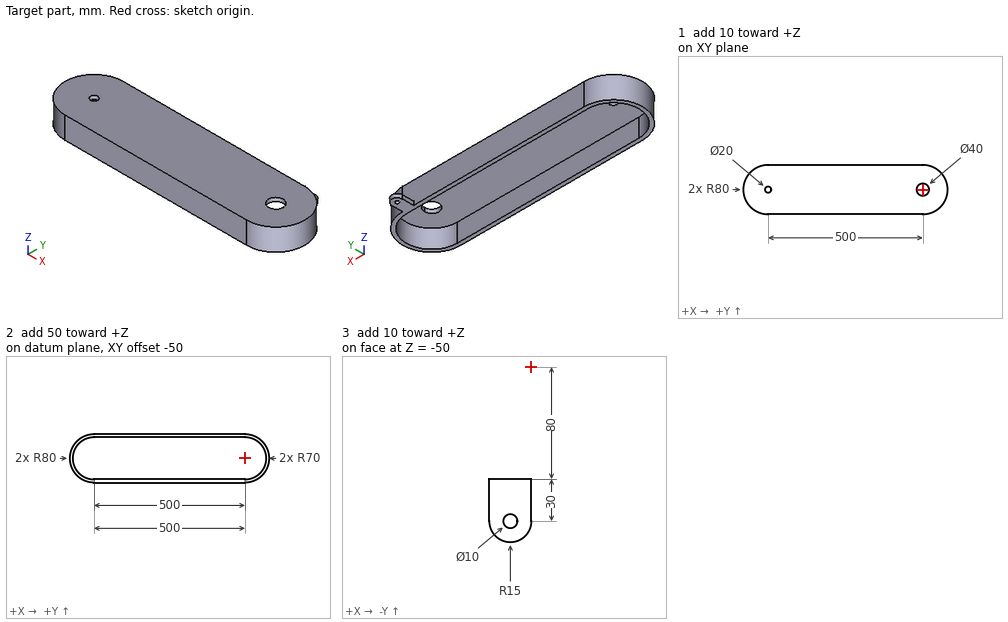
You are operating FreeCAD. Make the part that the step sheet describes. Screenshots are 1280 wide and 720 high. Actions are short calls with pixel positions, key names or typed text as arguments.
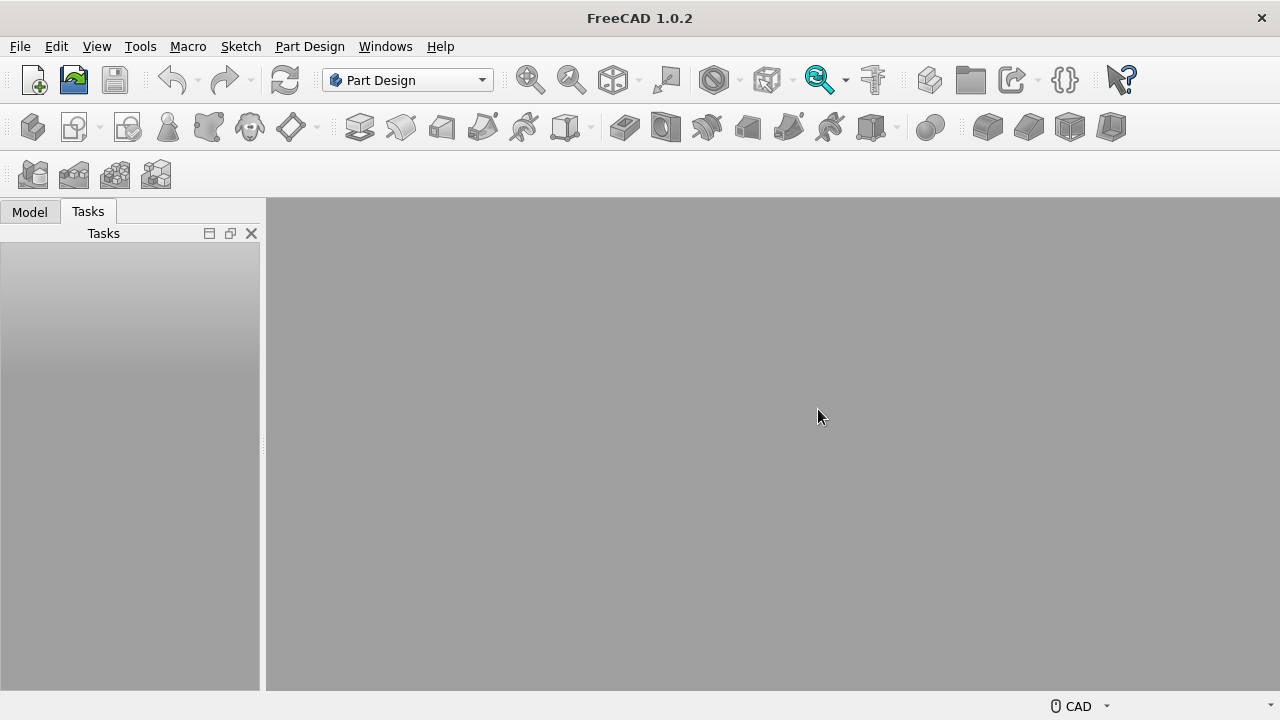
key(ctrl+n)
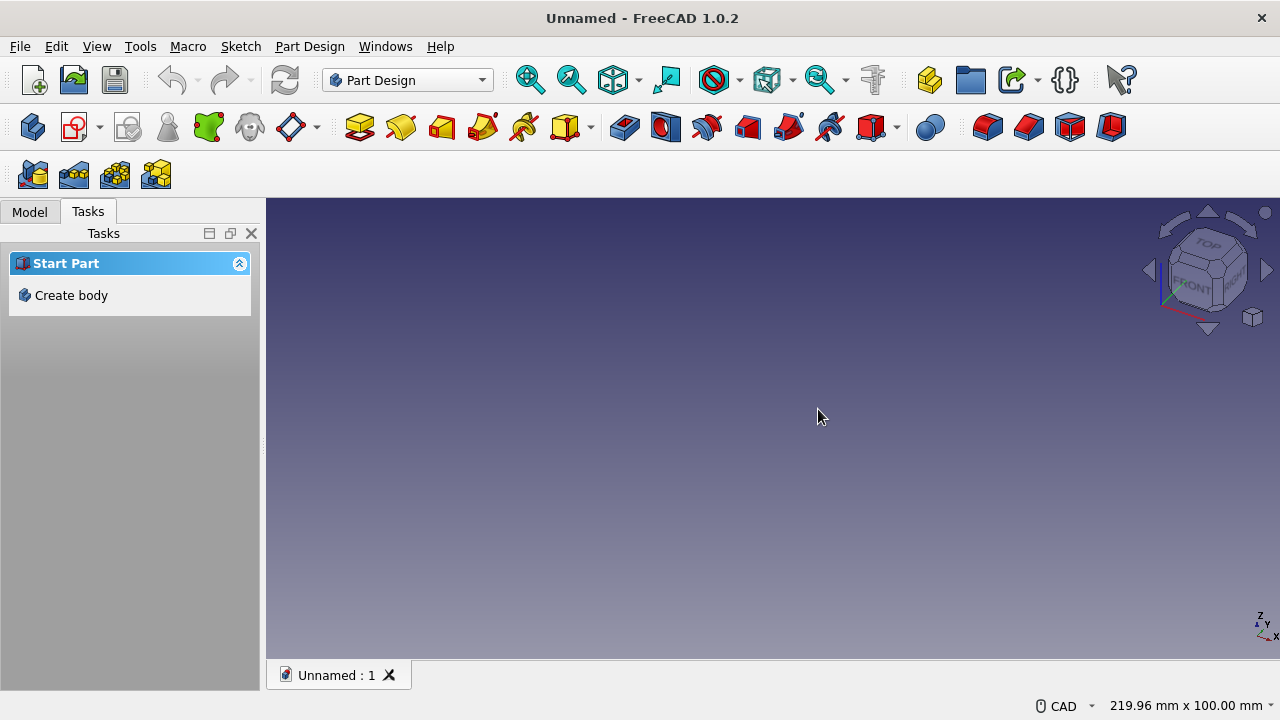
click(74, 128)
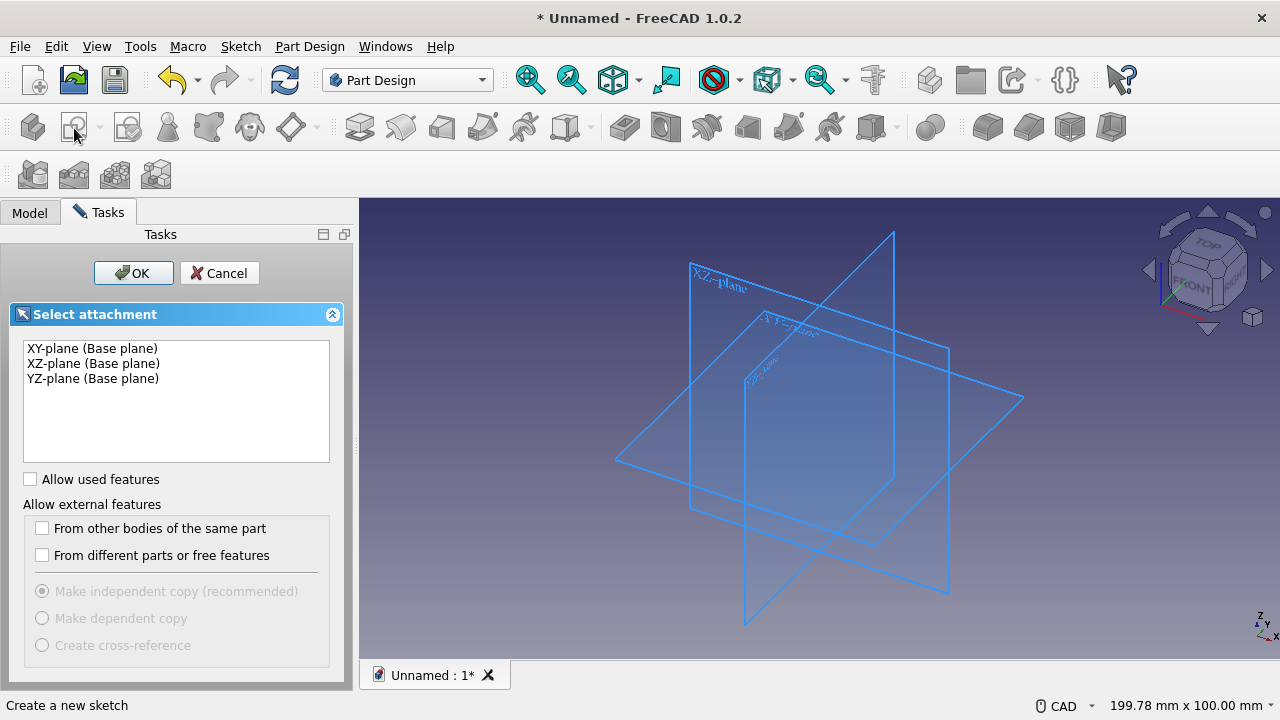
click(84, 348)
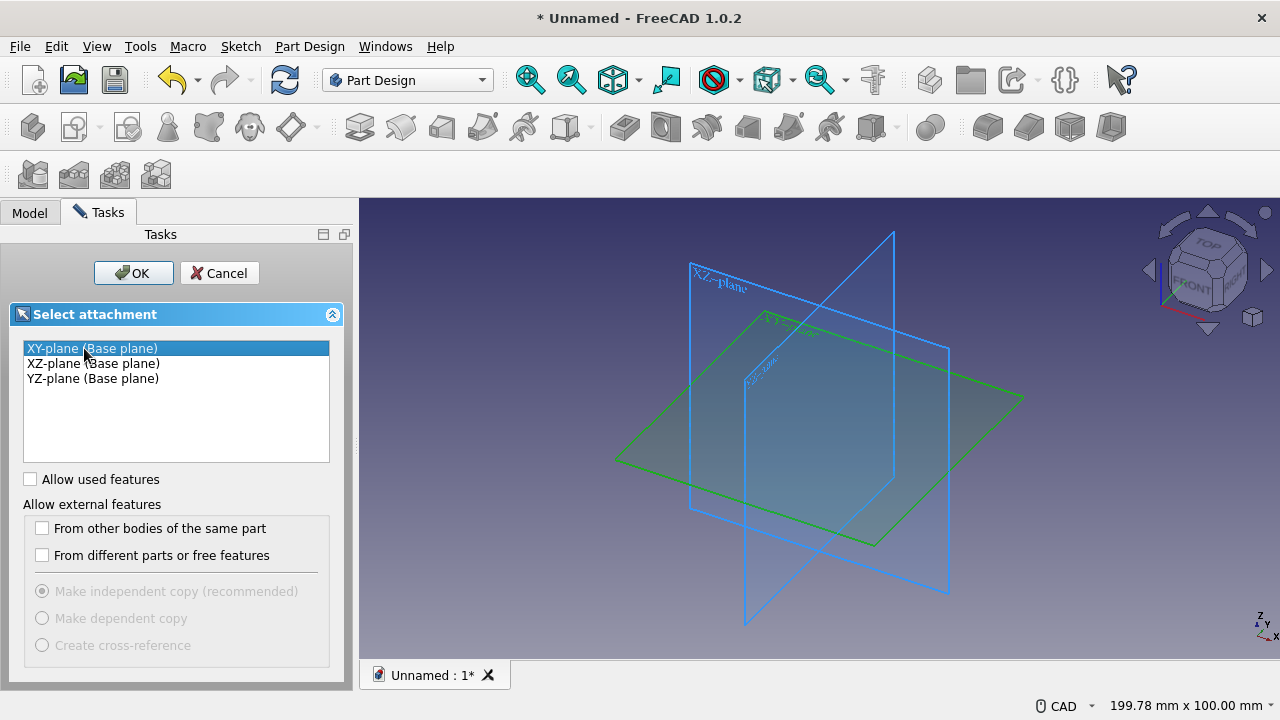
click(134, 273)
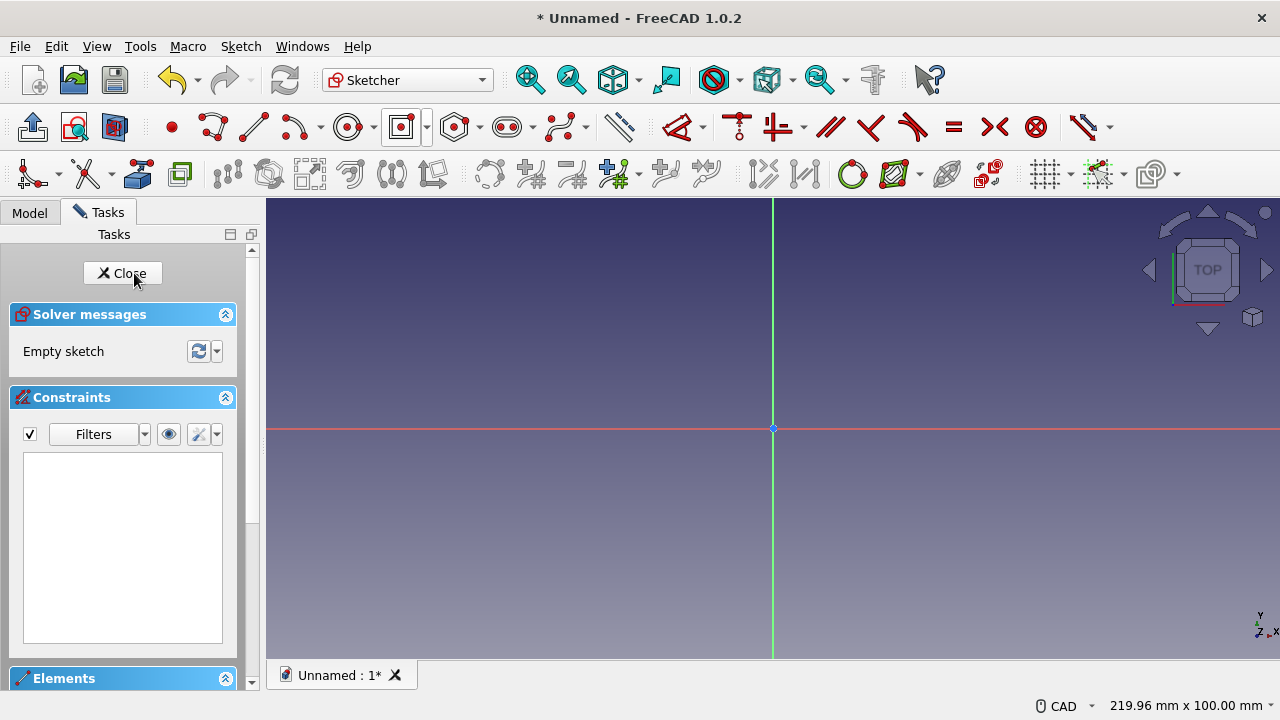
scroll(979, 428, down, 8)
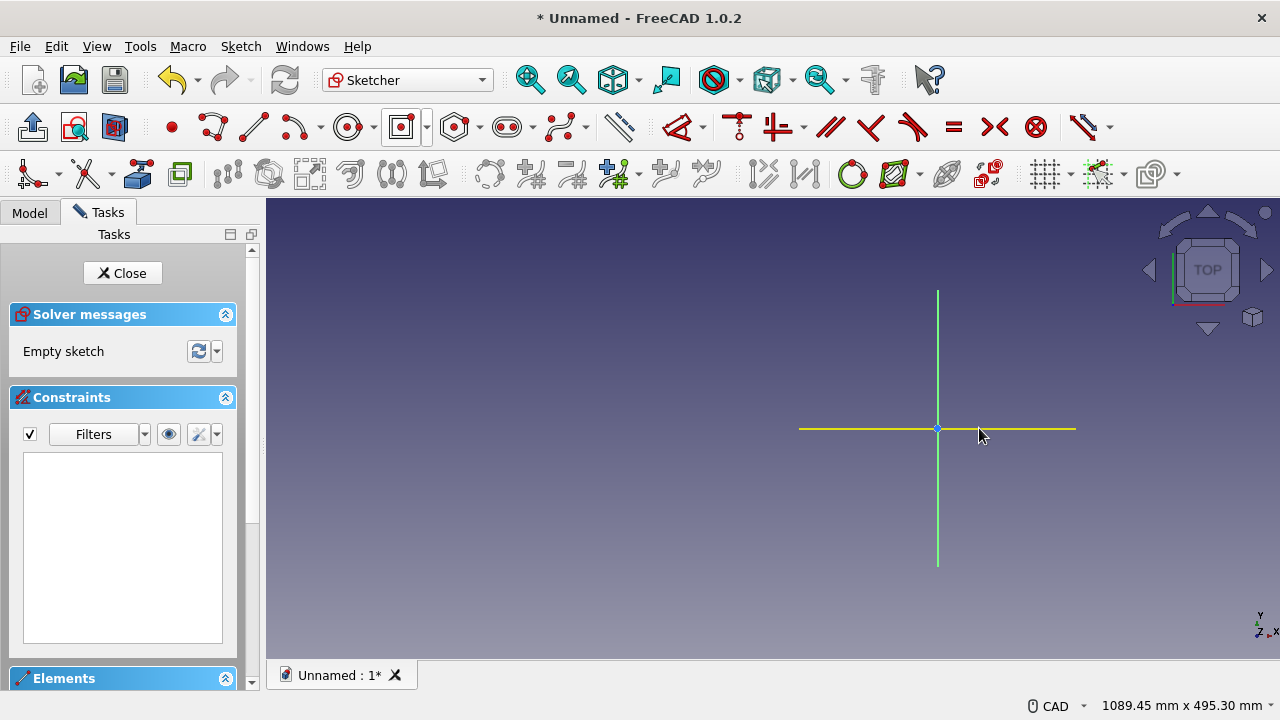
key(g)
key(s)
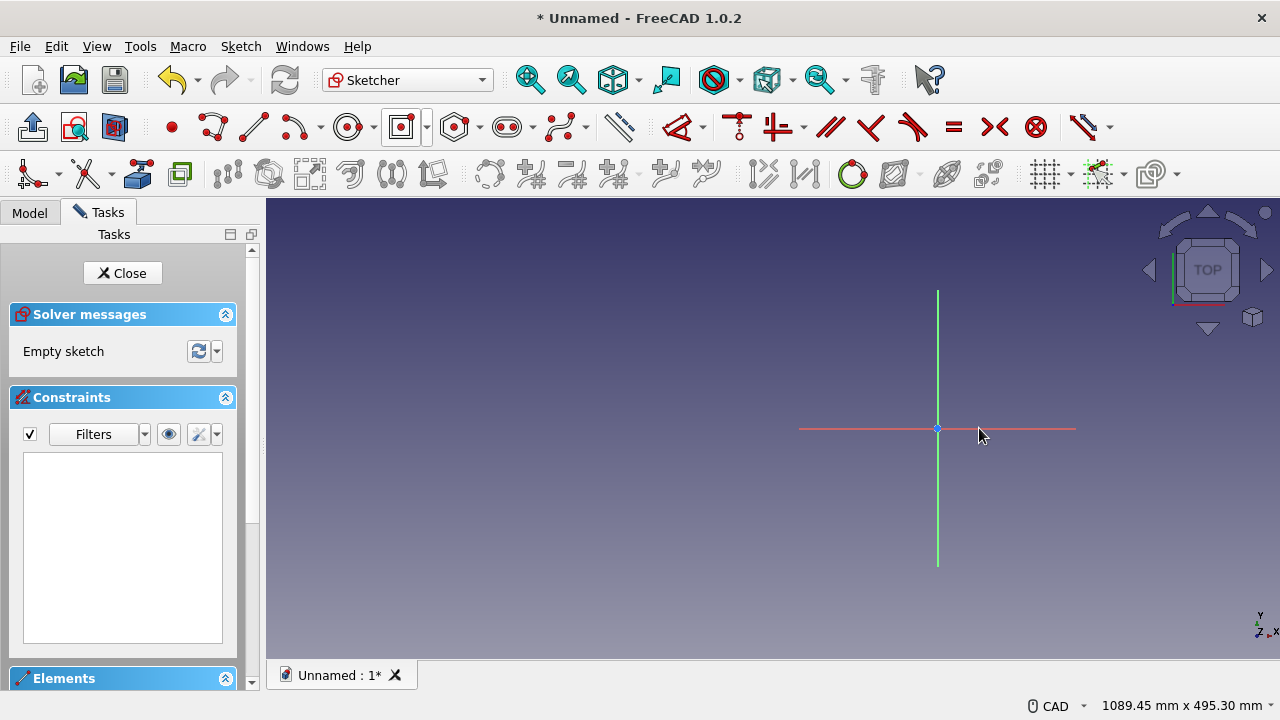
click(938, 428)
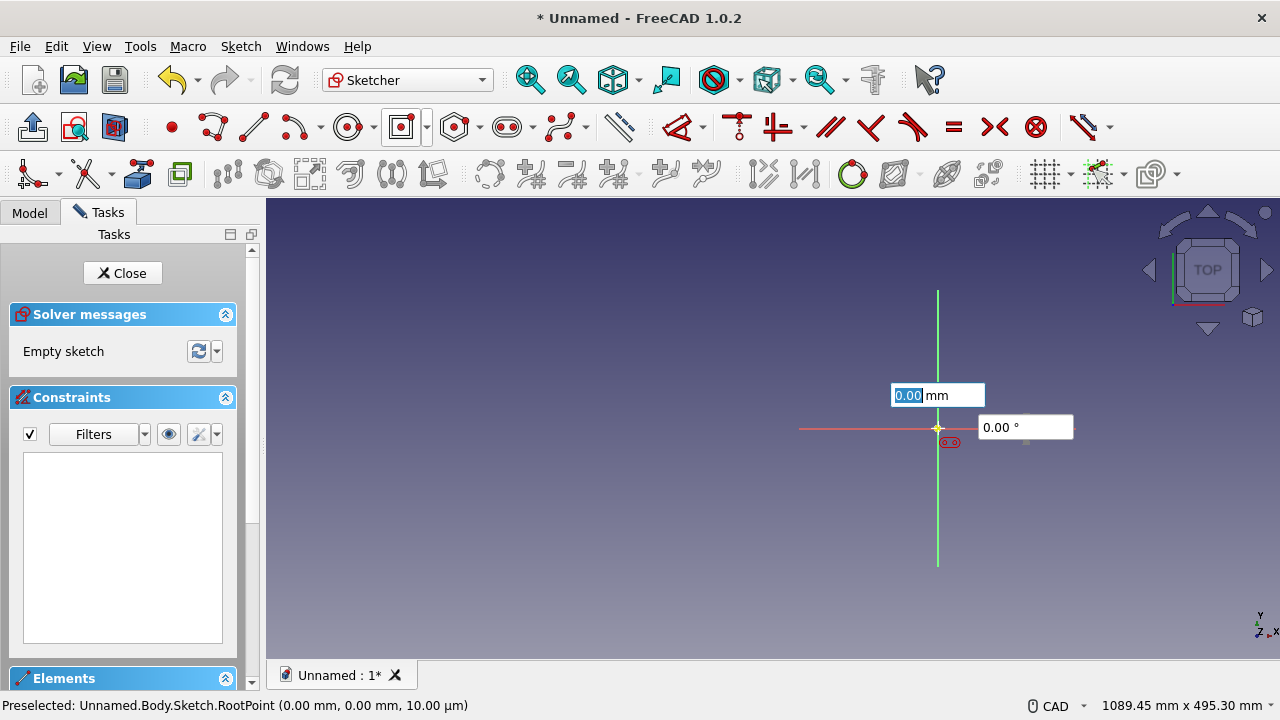
click(473, 420)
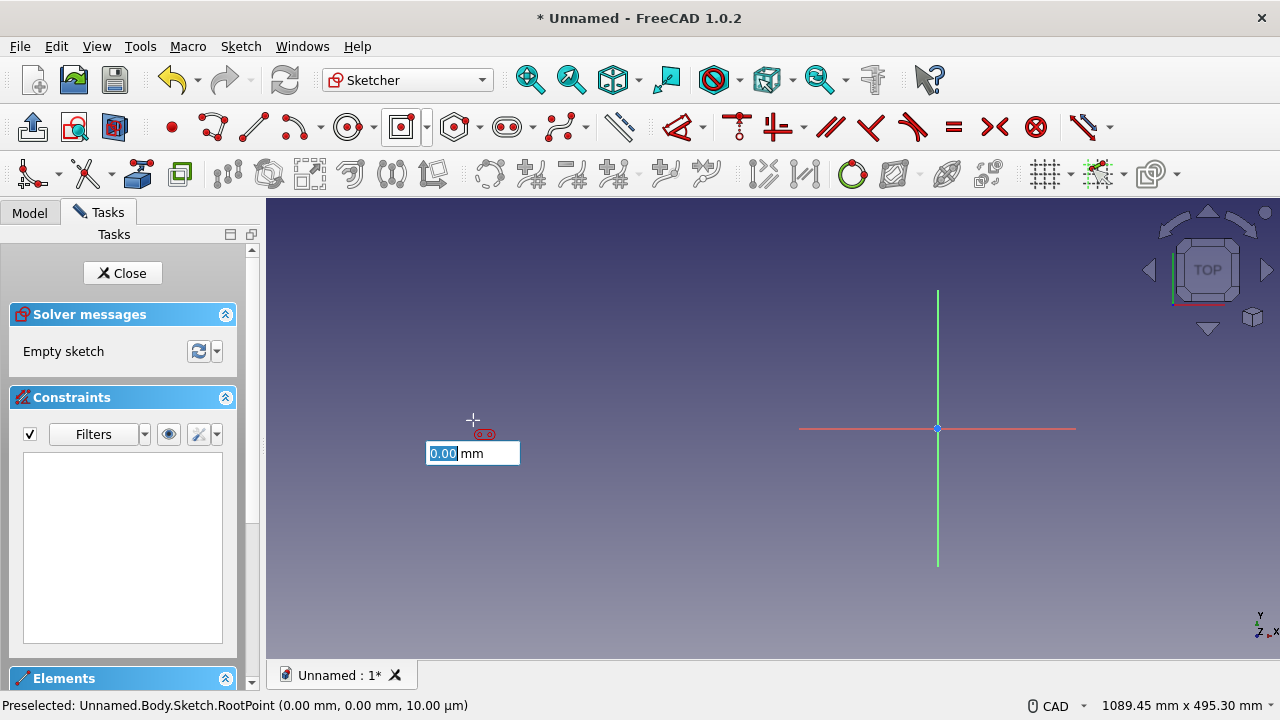
click(705, 354)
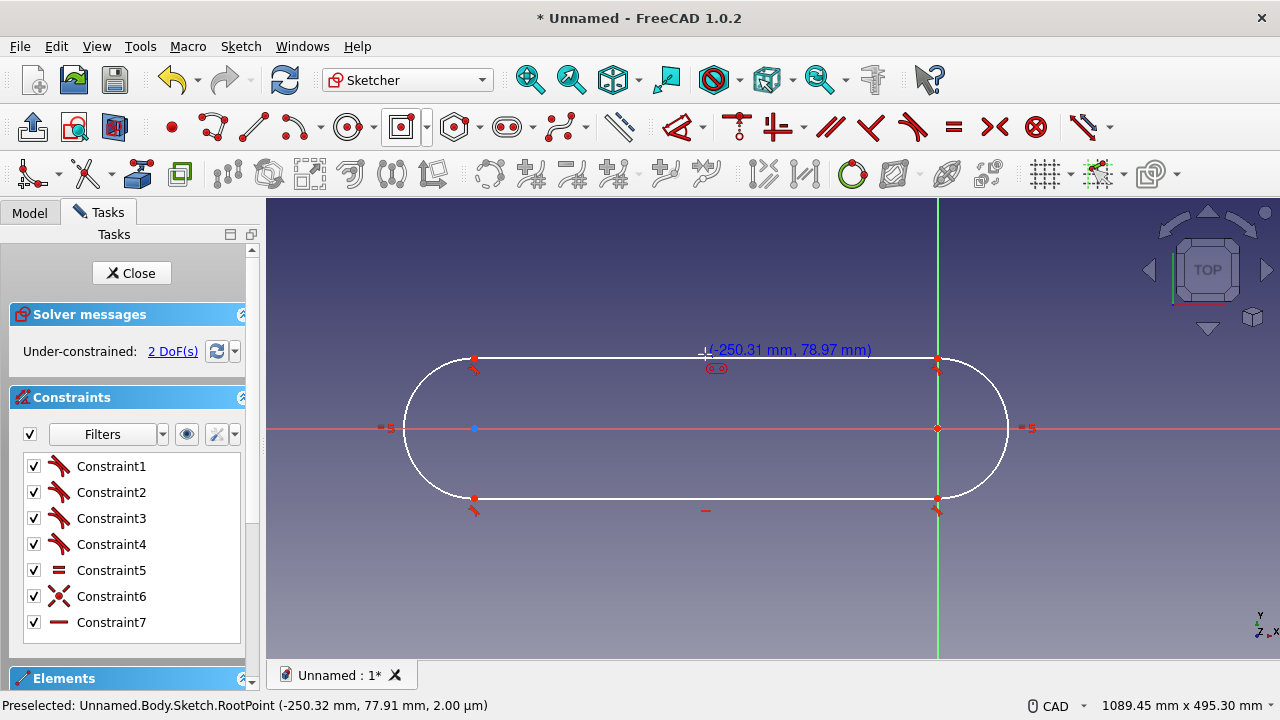
click(348, 128)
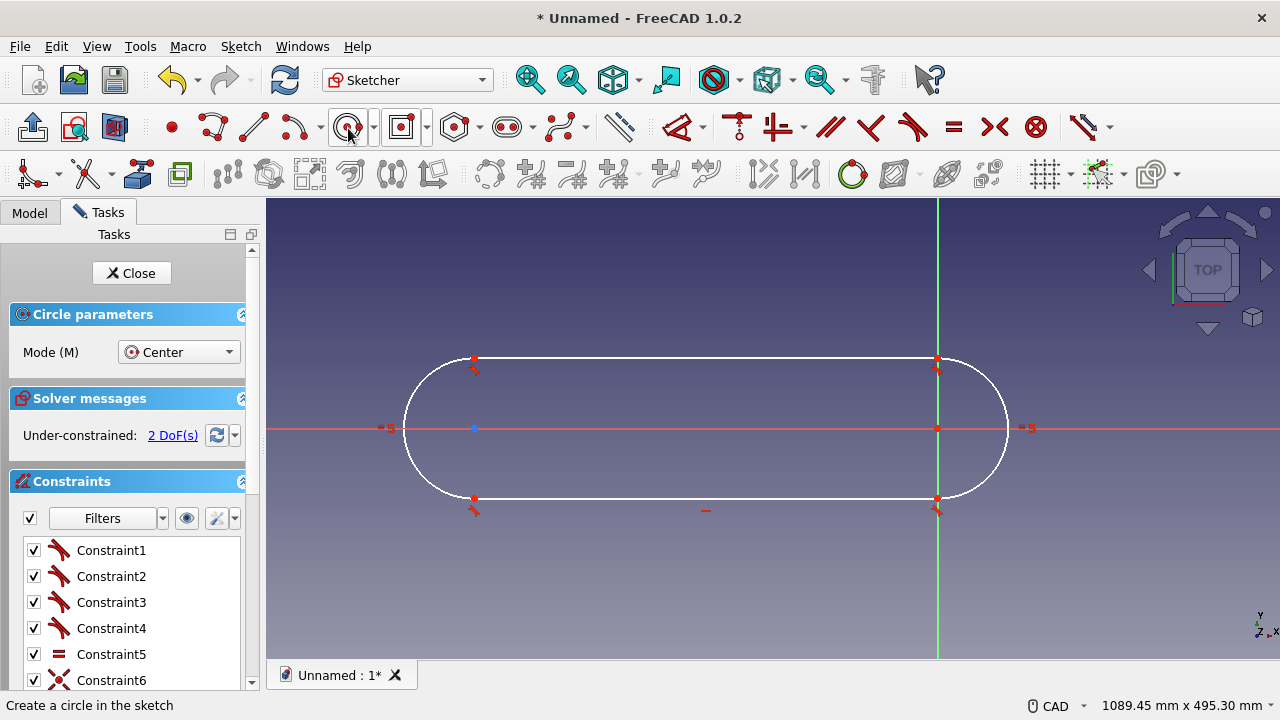
scroll(473, 428, up, 5)